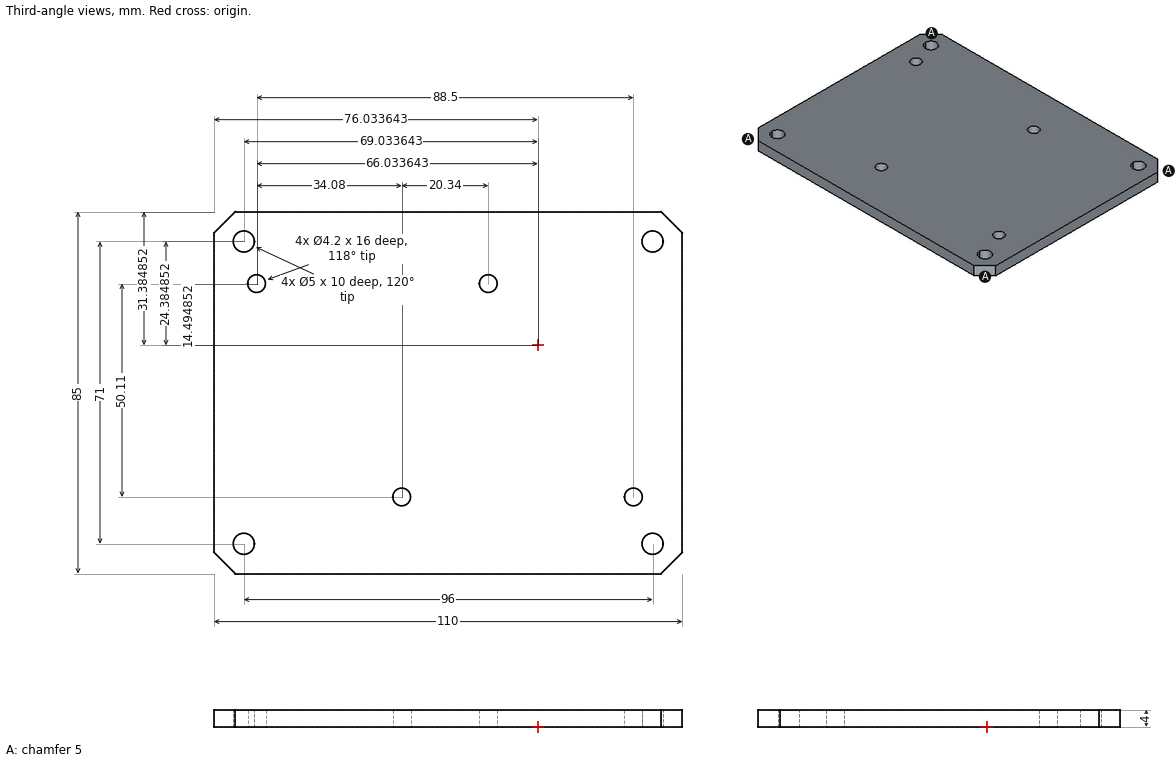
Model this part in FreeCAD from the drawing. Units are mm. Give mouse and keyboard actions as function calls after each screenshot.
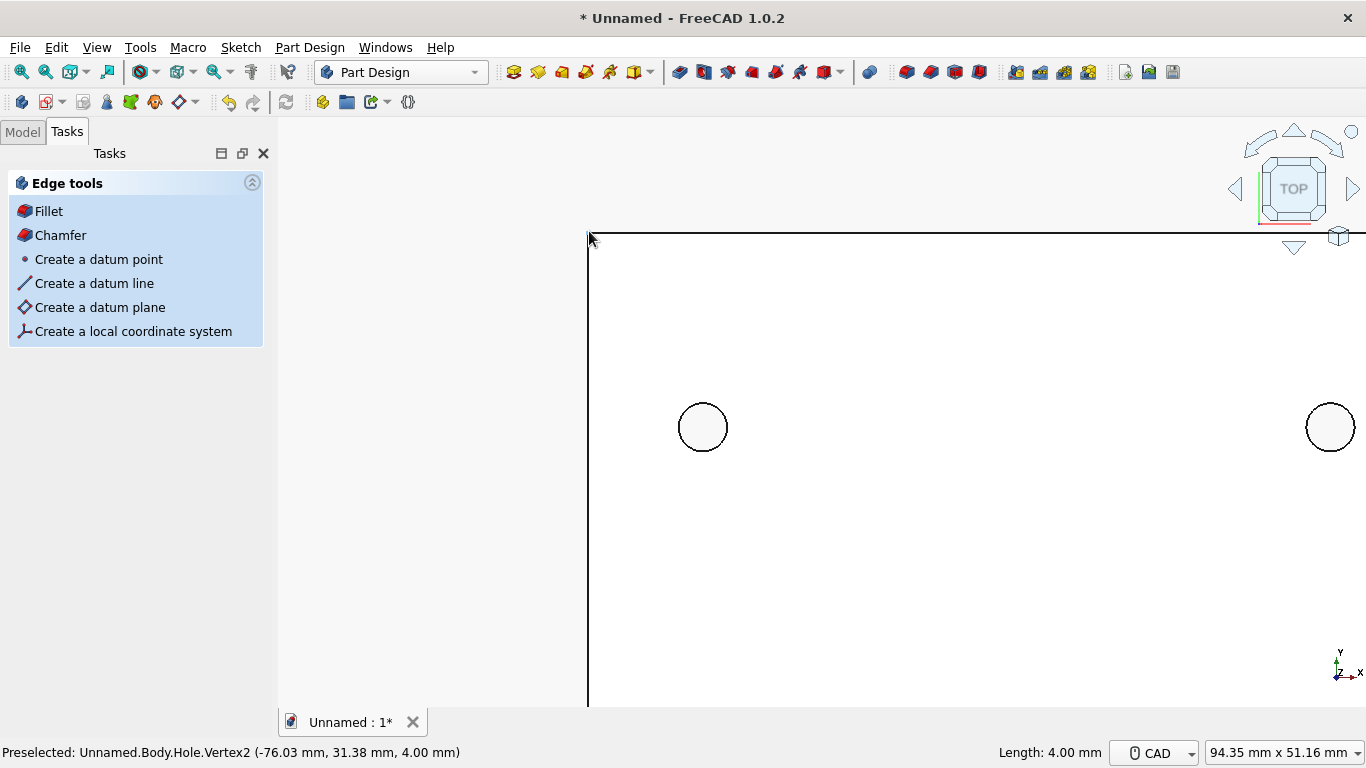
click(22, 72)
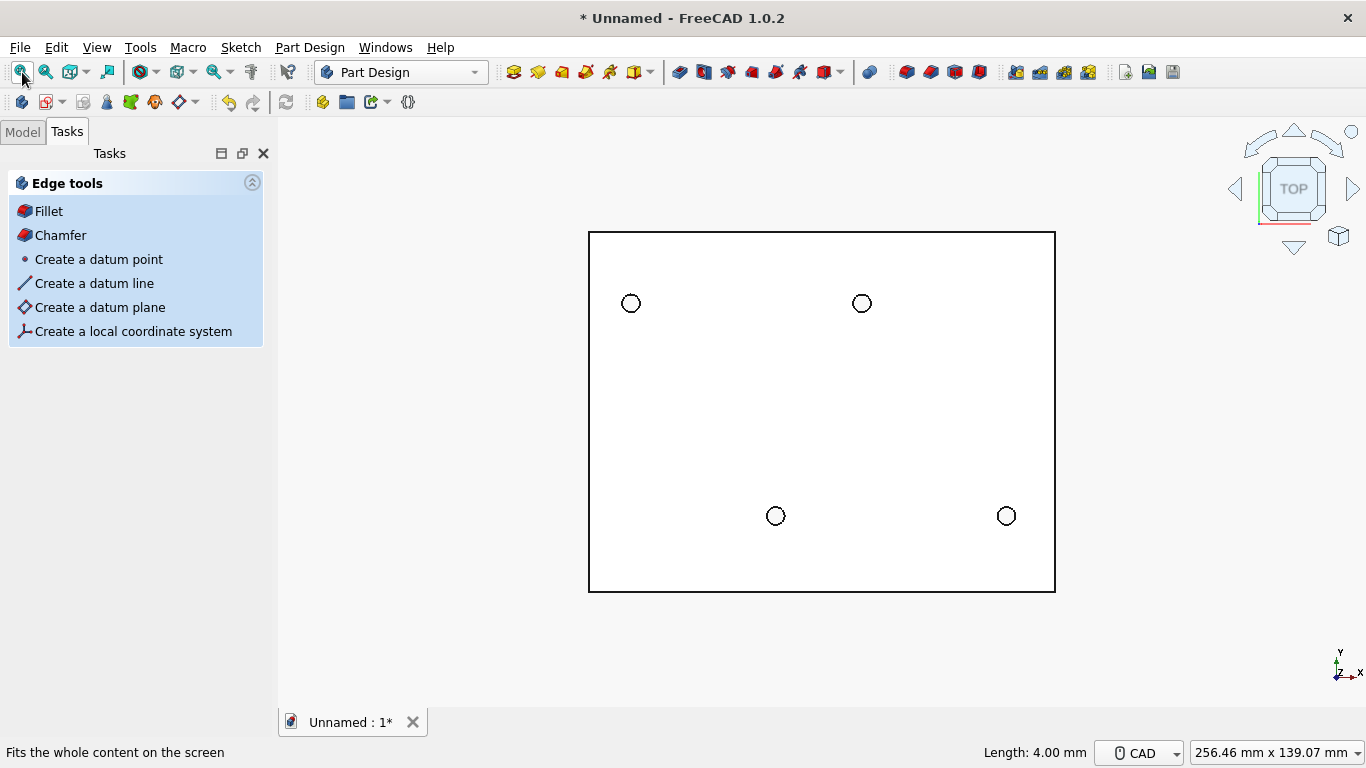
key(1)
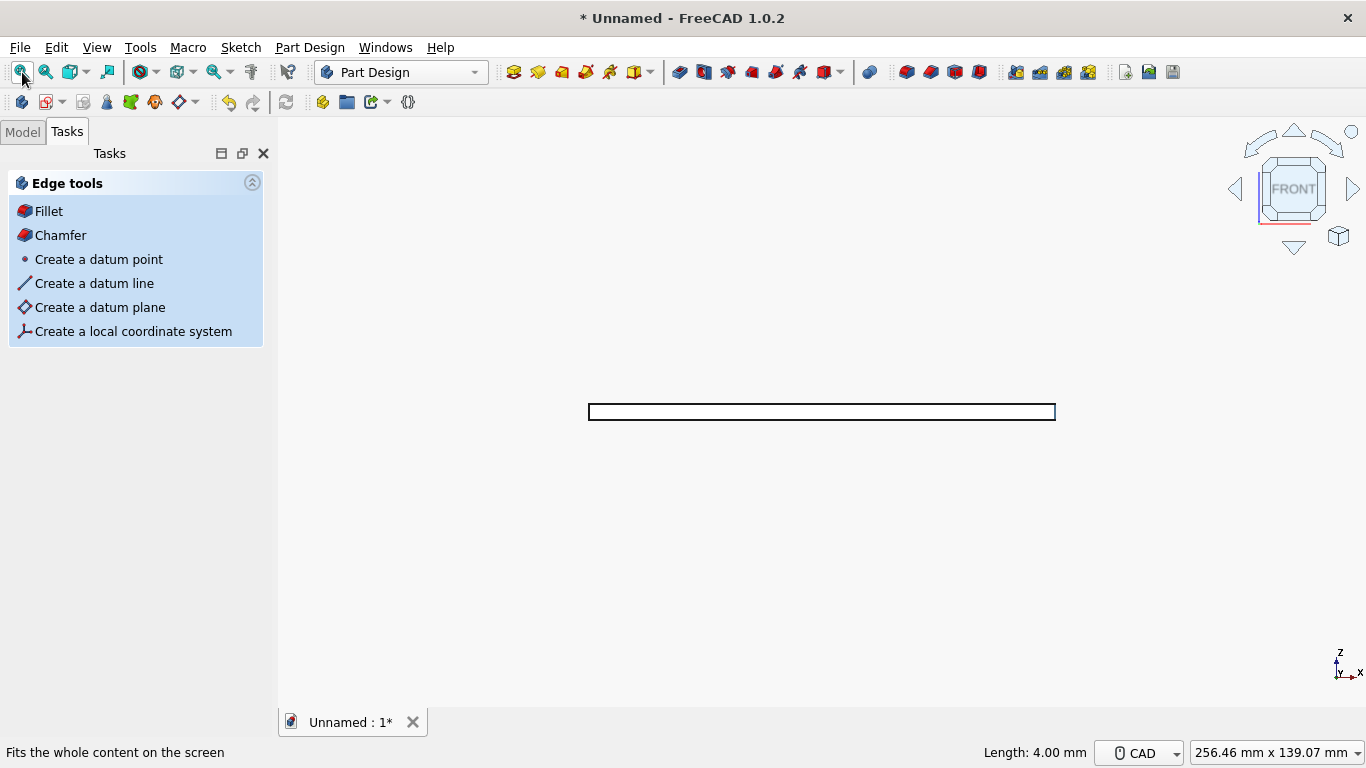
click(22, 72)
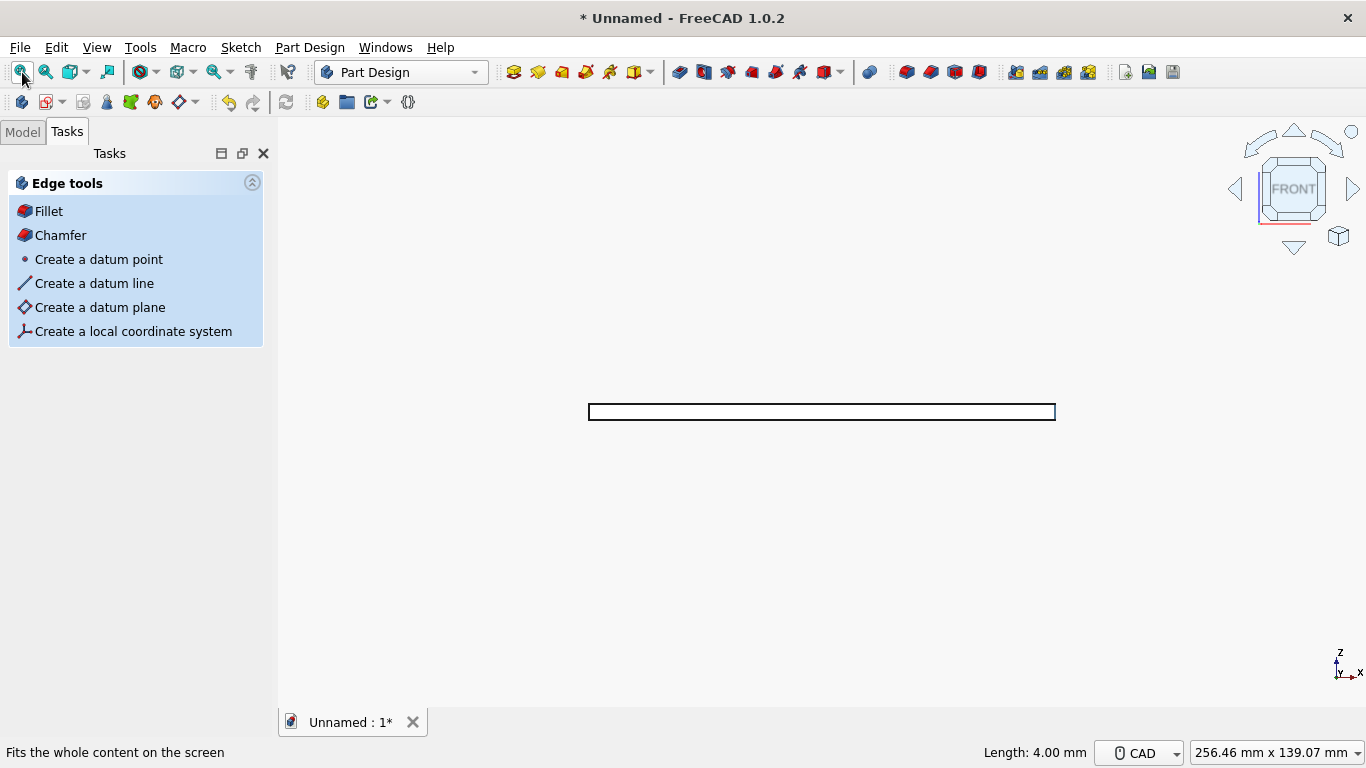
click(589, 411, ctrl)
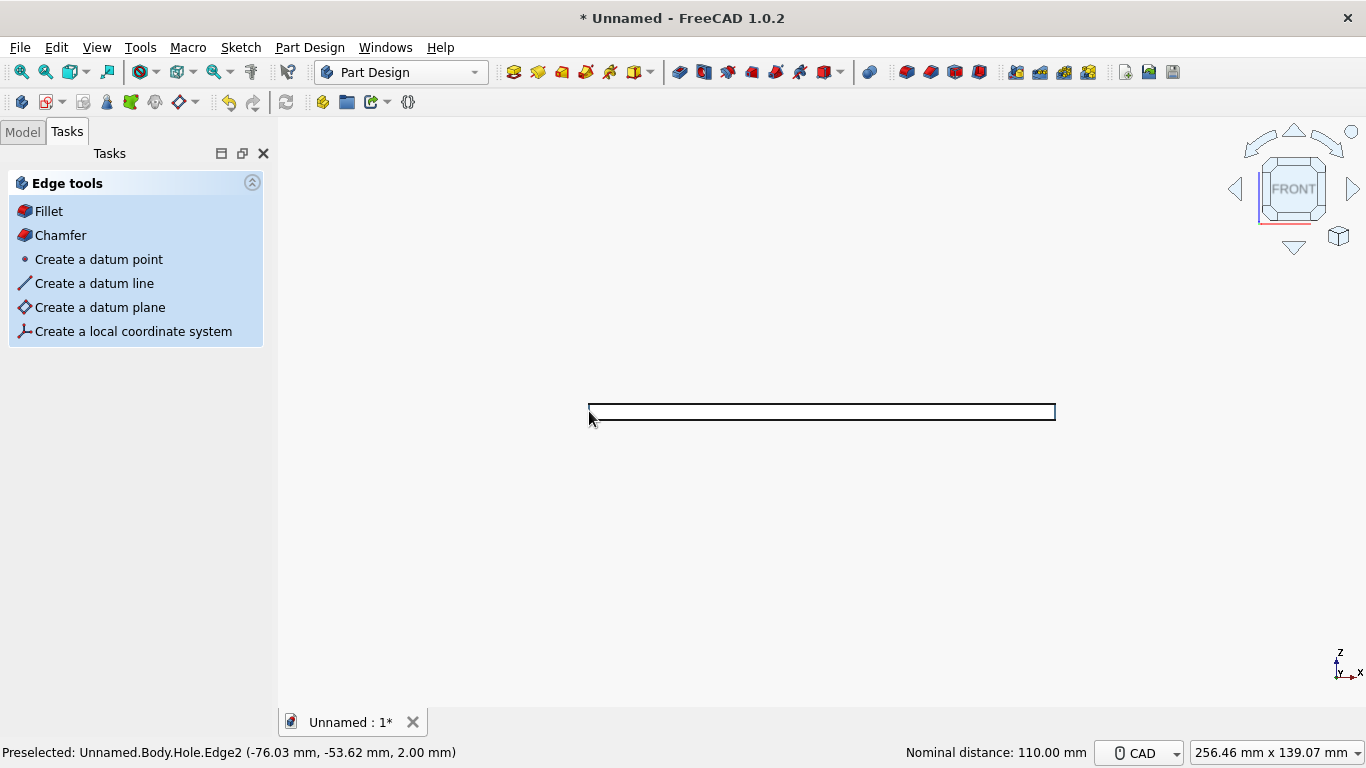
scroll(589, 411, up, 5)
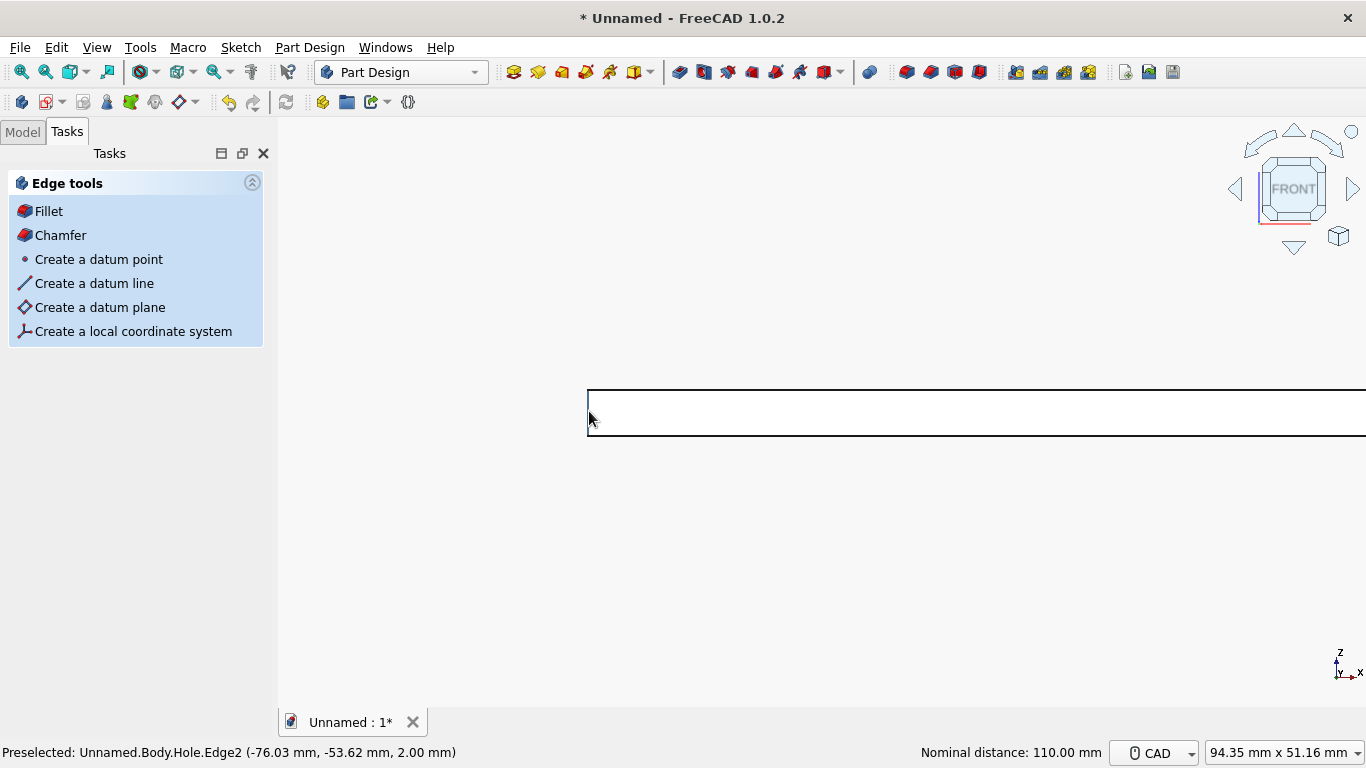
click(22, 72)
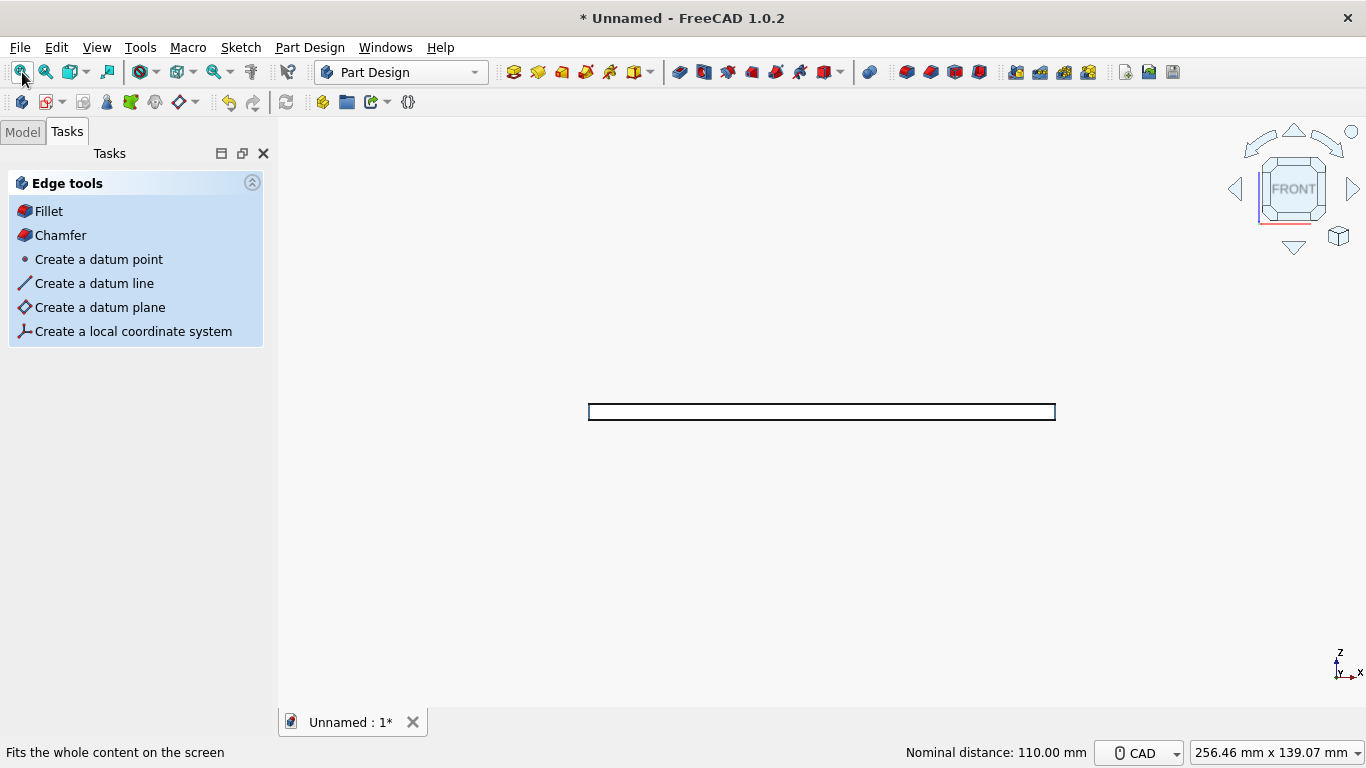
key(3)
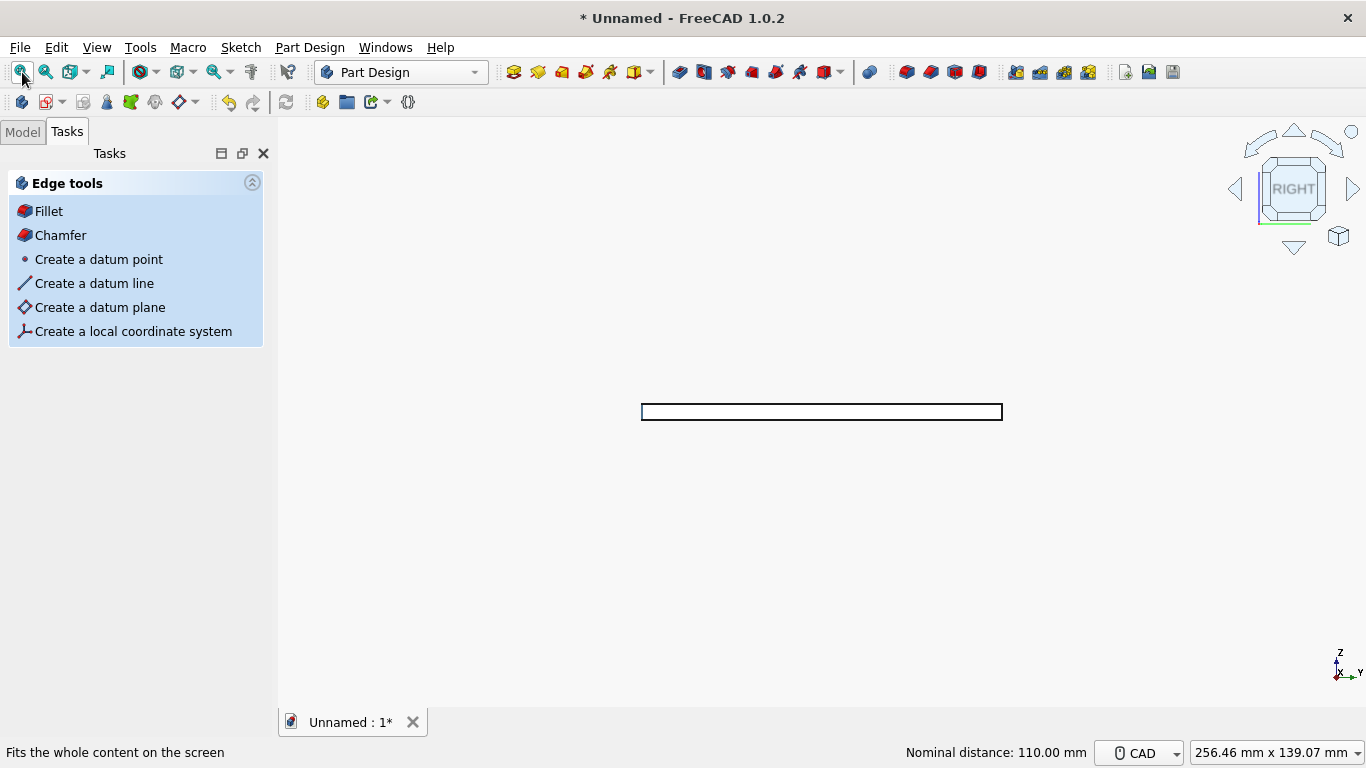
click(22, 72)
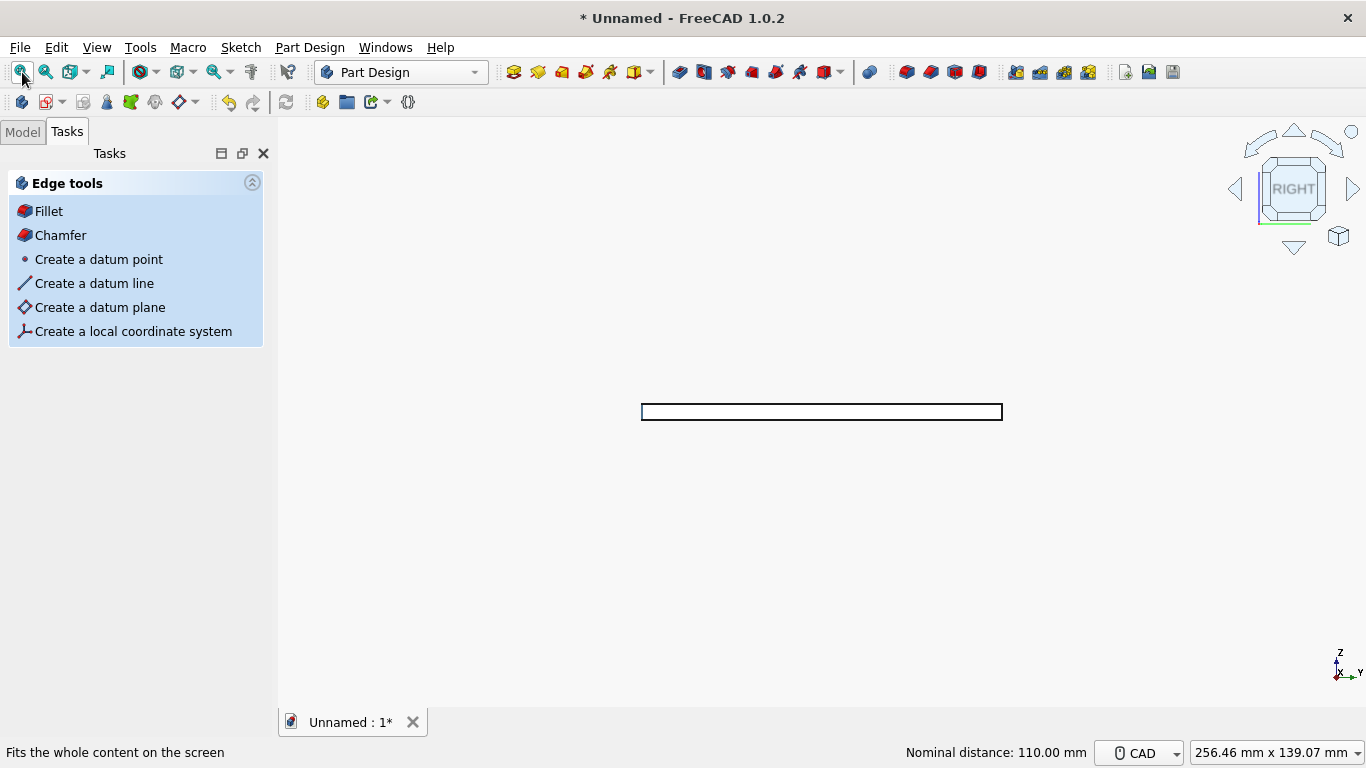
click(1002, 411, ctrl)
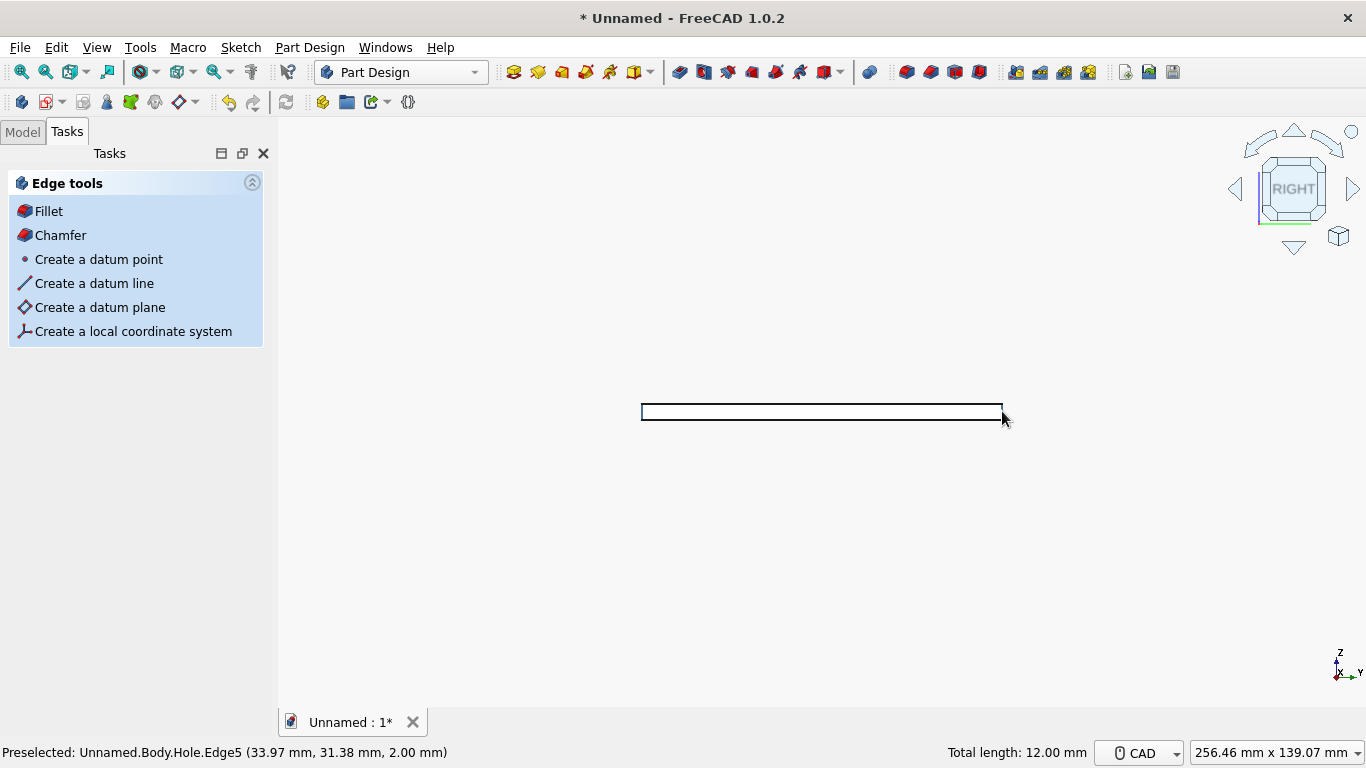
scroll(1002, 411, up, 5)